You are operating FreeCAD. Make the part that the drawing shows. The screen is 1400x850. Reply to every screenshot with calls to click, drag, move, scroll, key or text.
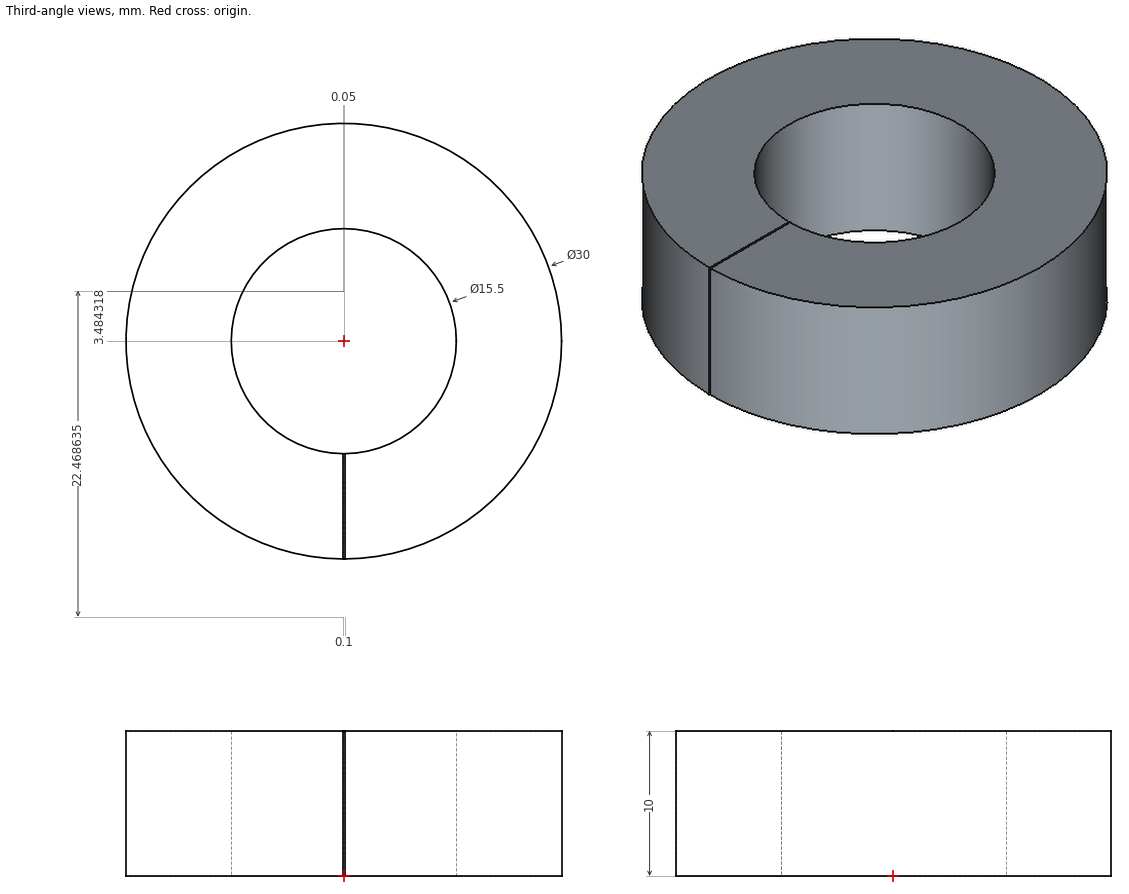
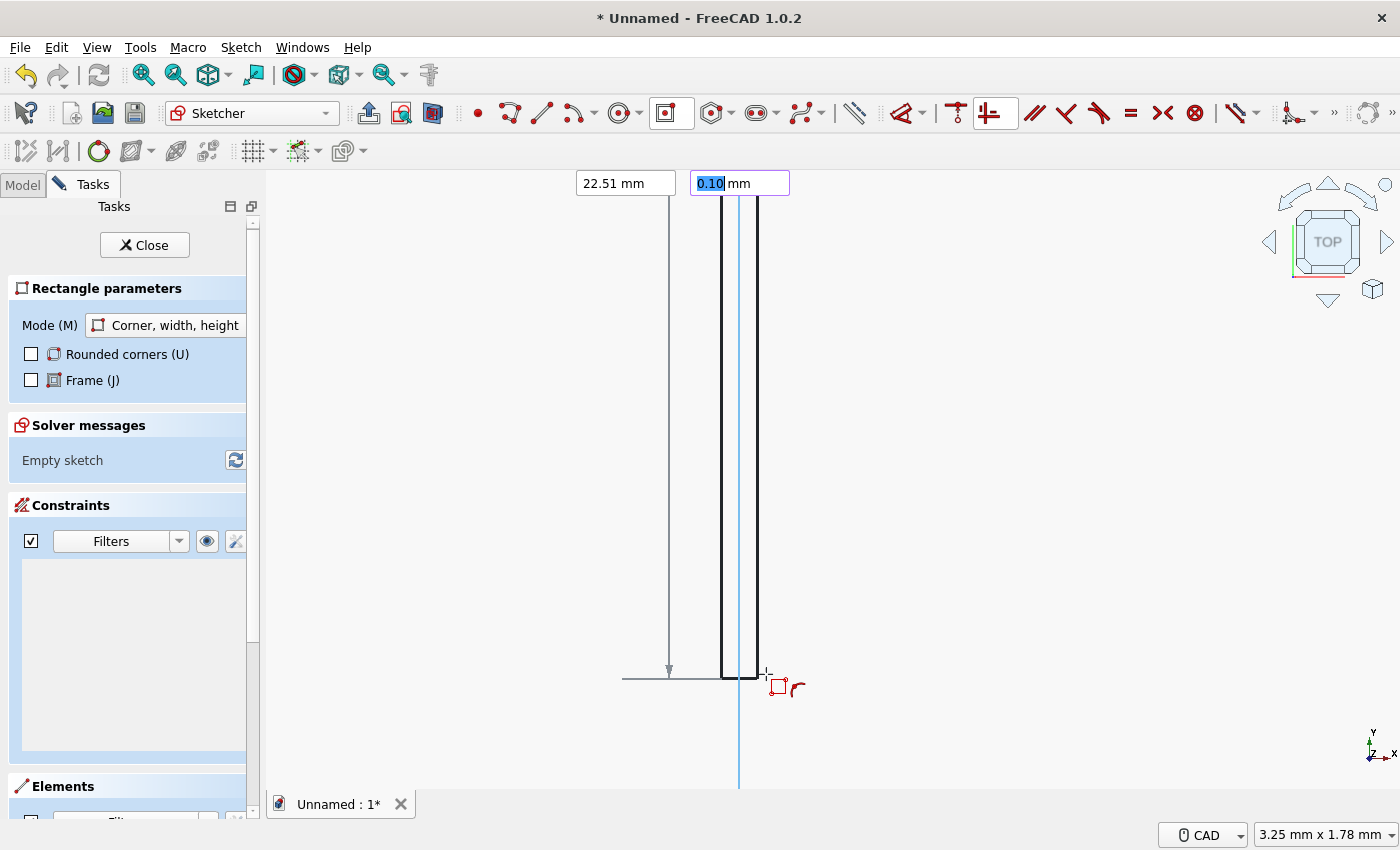
click(756, 663)
key(Escape)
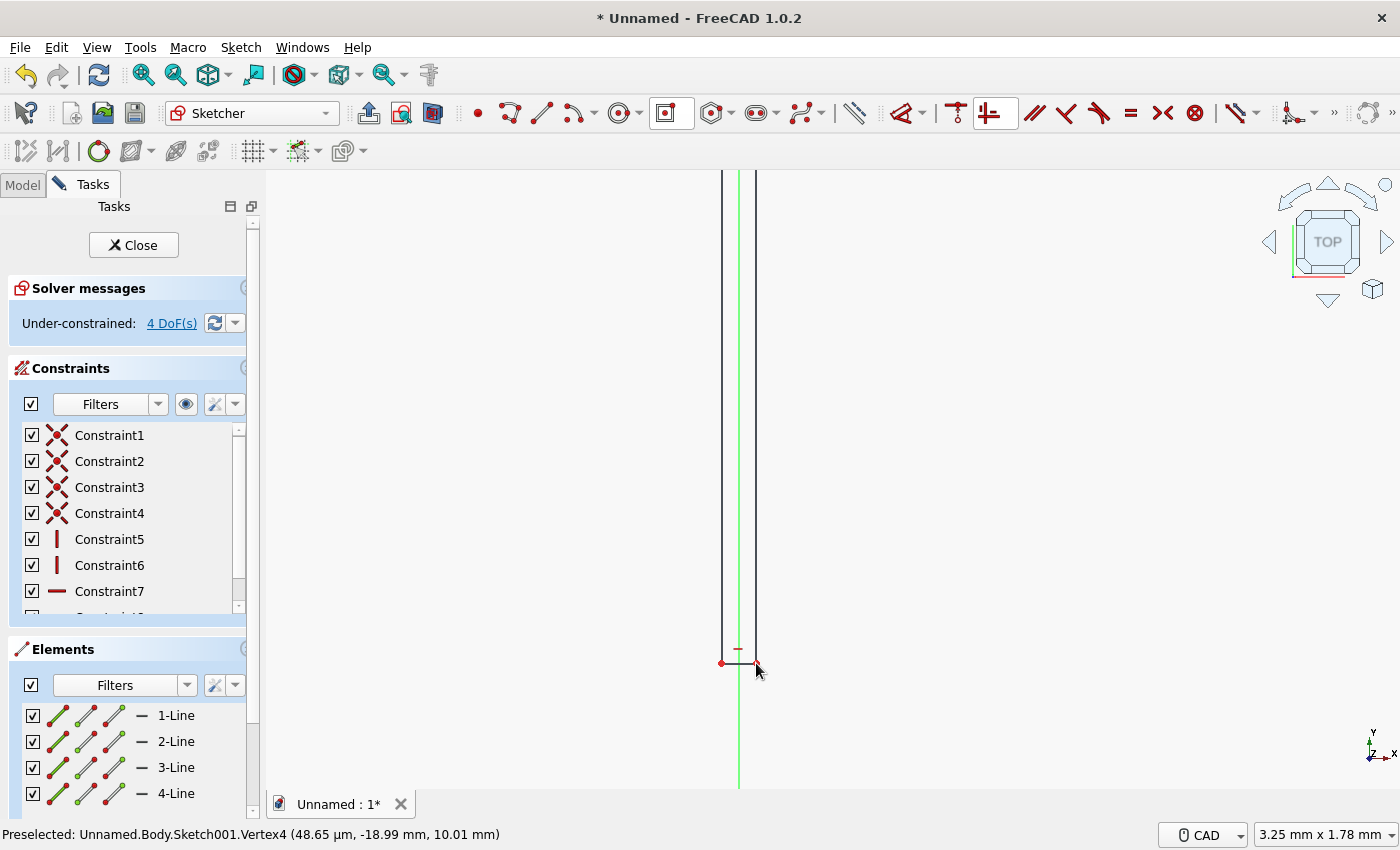
key(d)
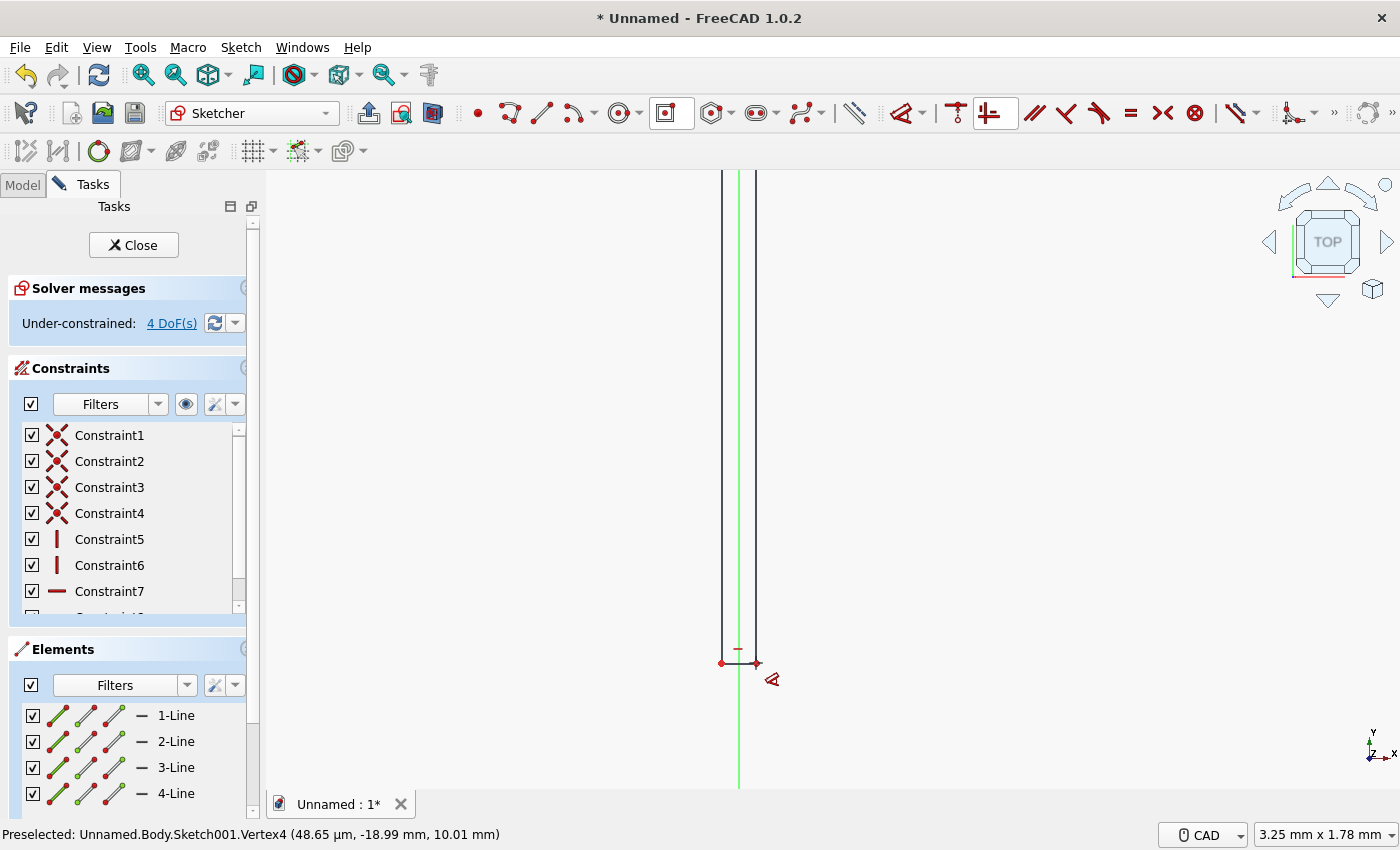
click(735, 664)
click(731, 698)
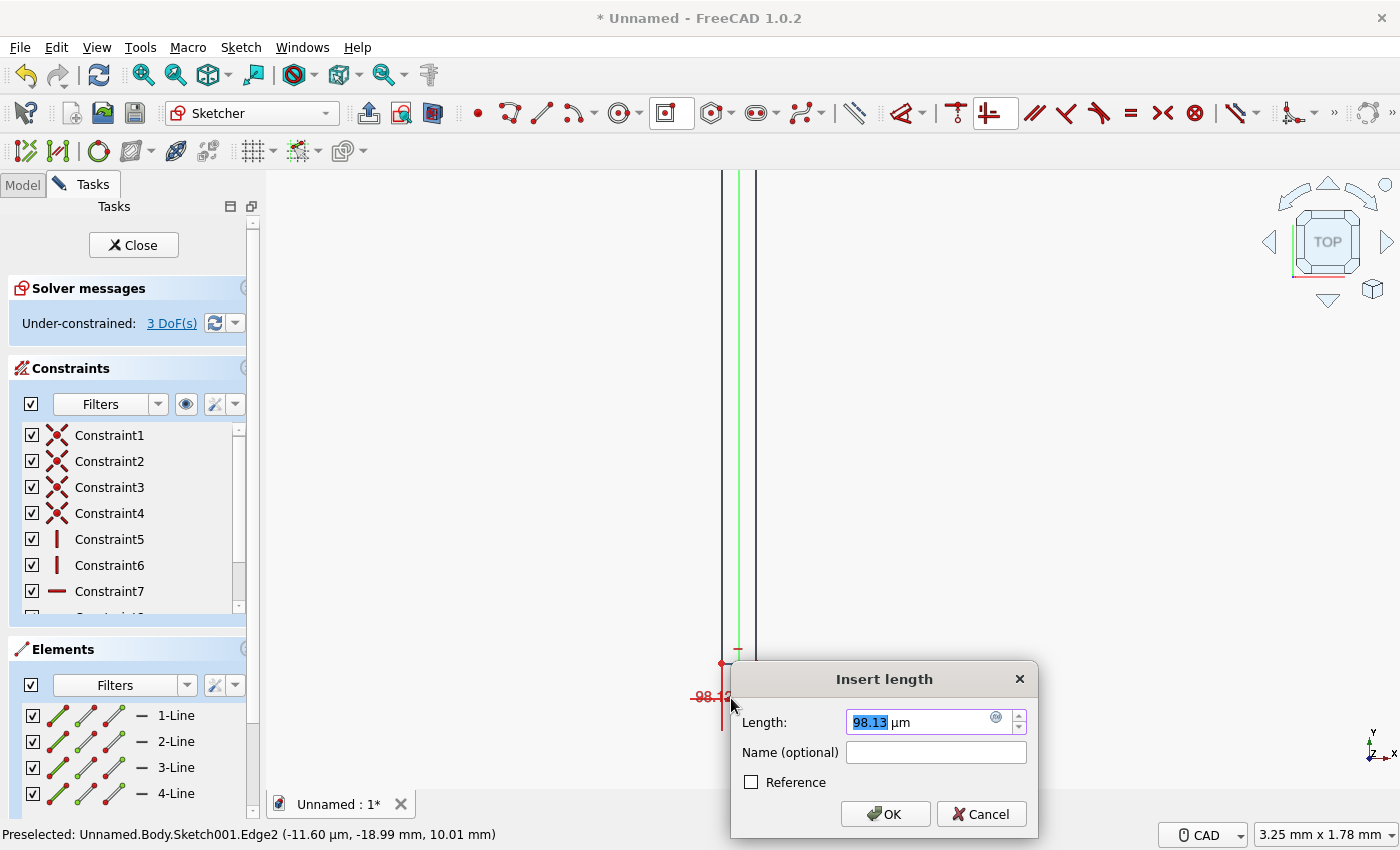
key(ctrl+a)
text(0.1 mm)
key(Return)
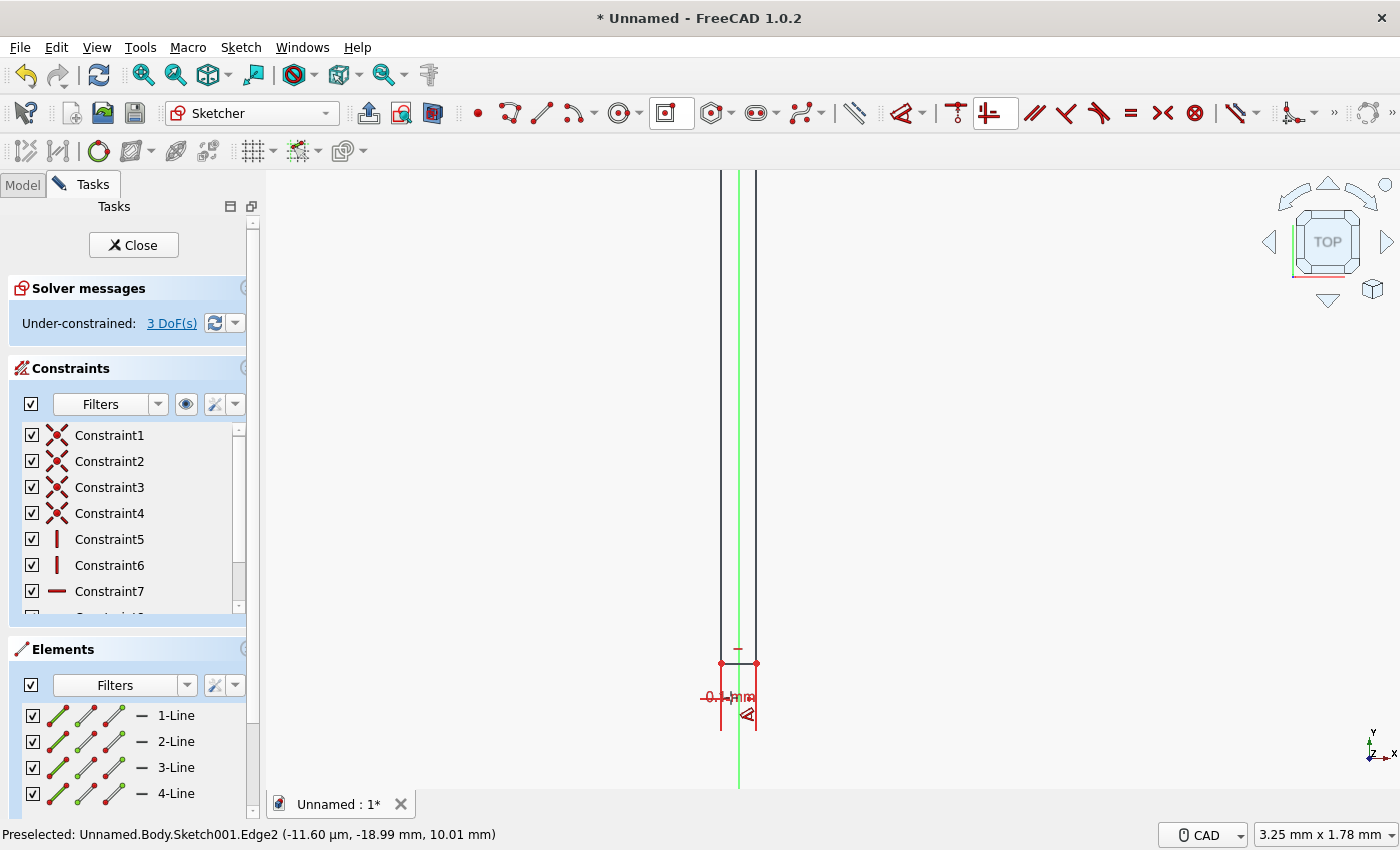
scroll(766, 675, down, 15)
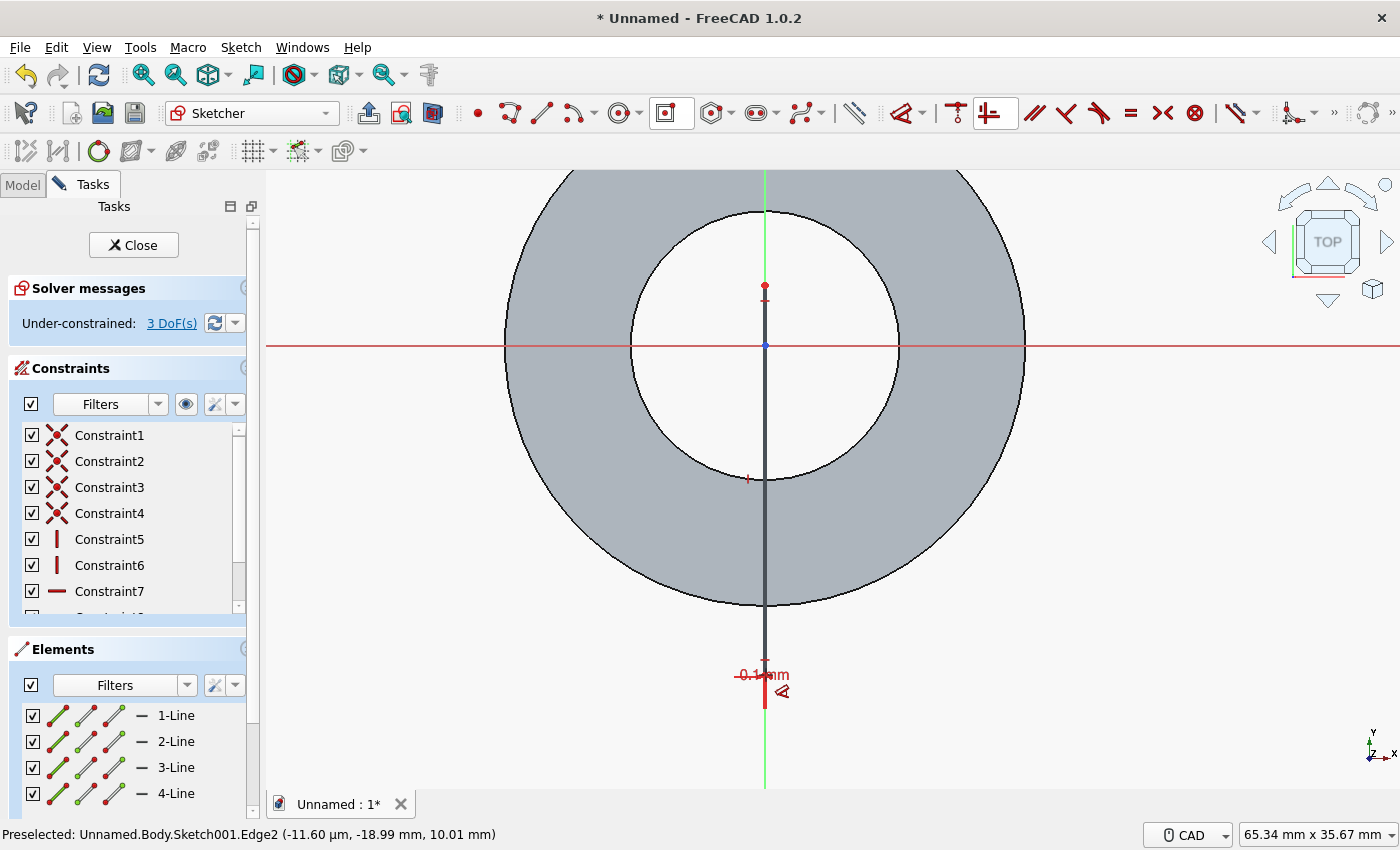
scroll(764, 285, up, 20)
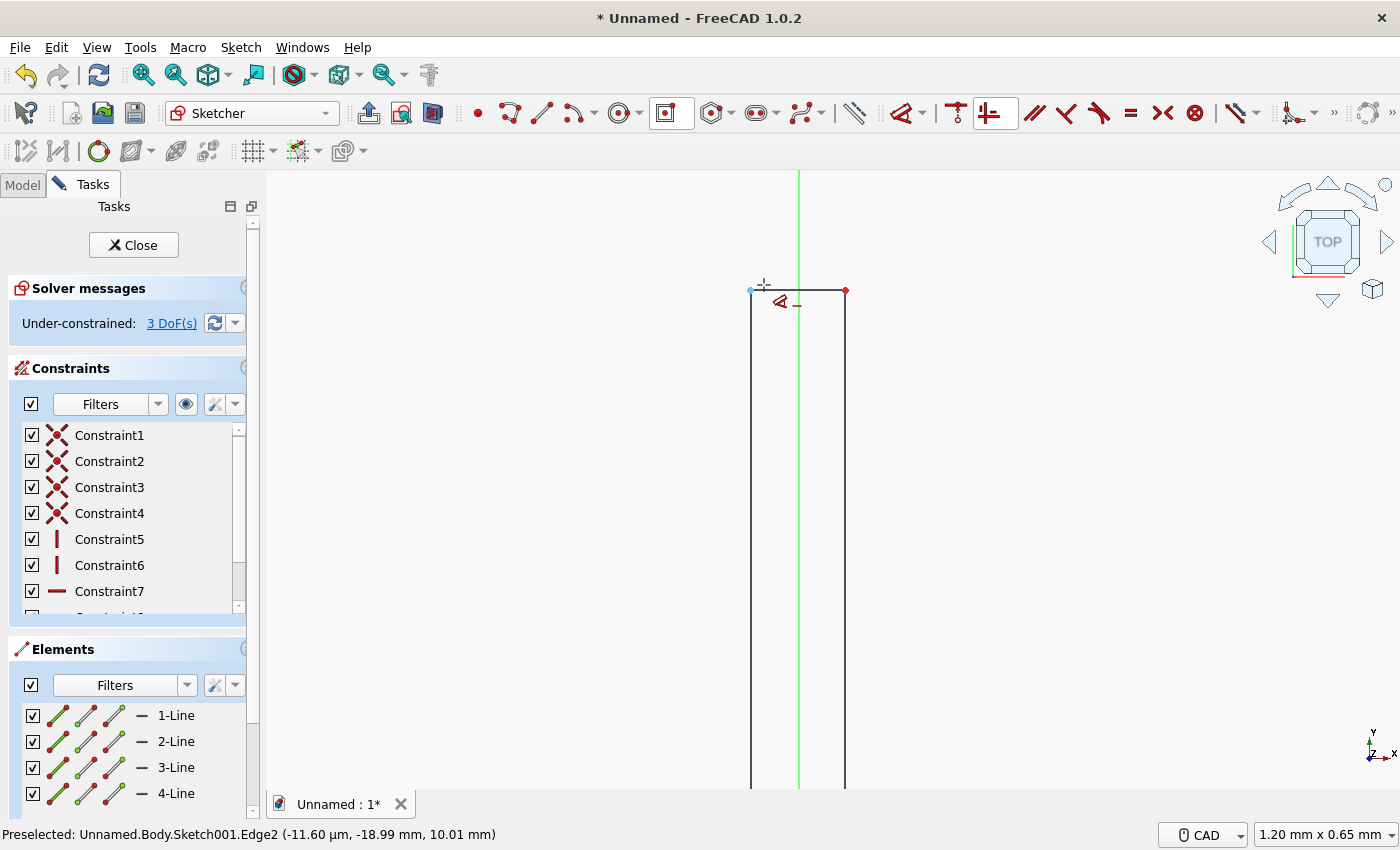
click(751, 290)
click(775, 256)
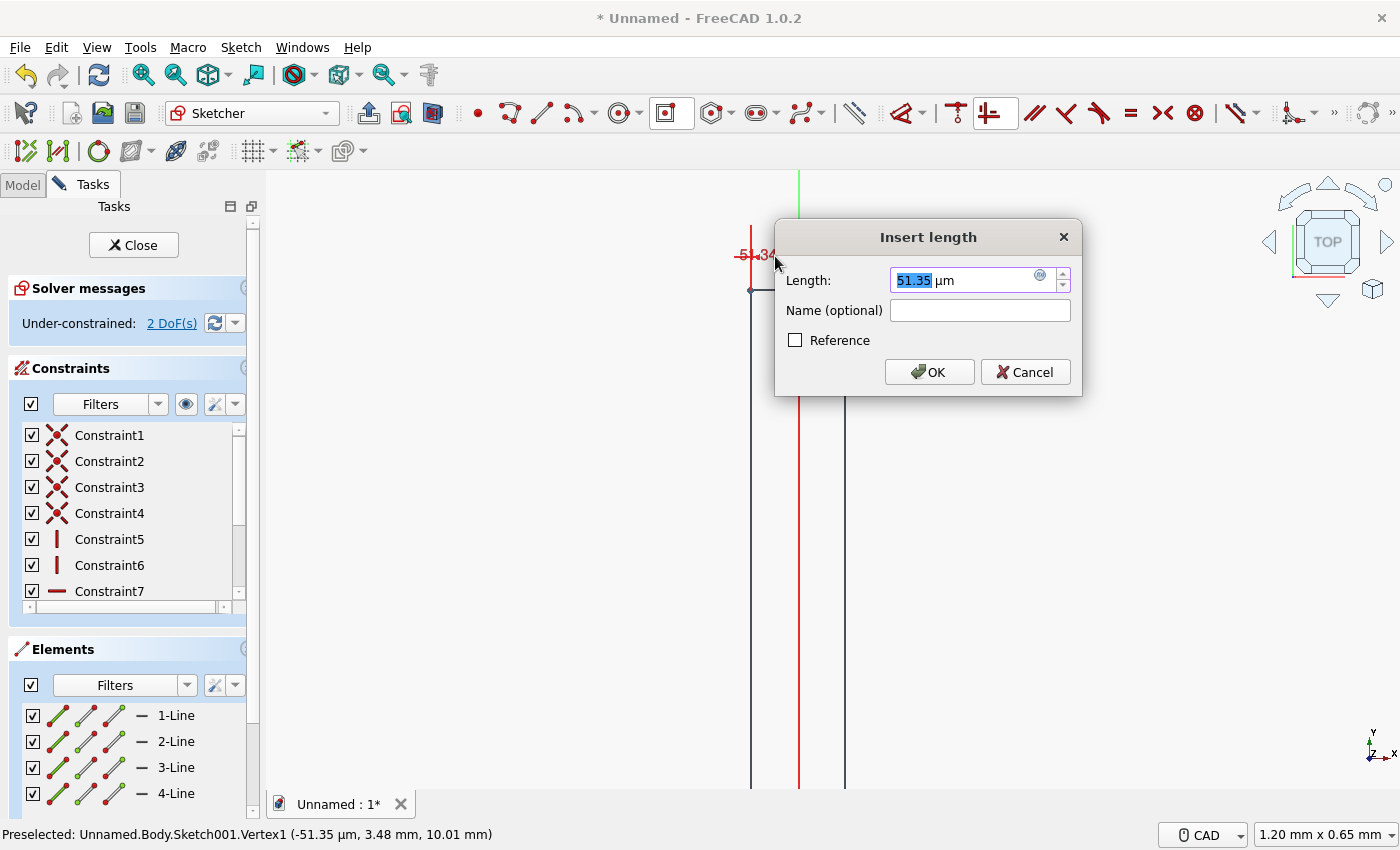
key(ctrl+a)
text(0.05 mm)
key(Return)